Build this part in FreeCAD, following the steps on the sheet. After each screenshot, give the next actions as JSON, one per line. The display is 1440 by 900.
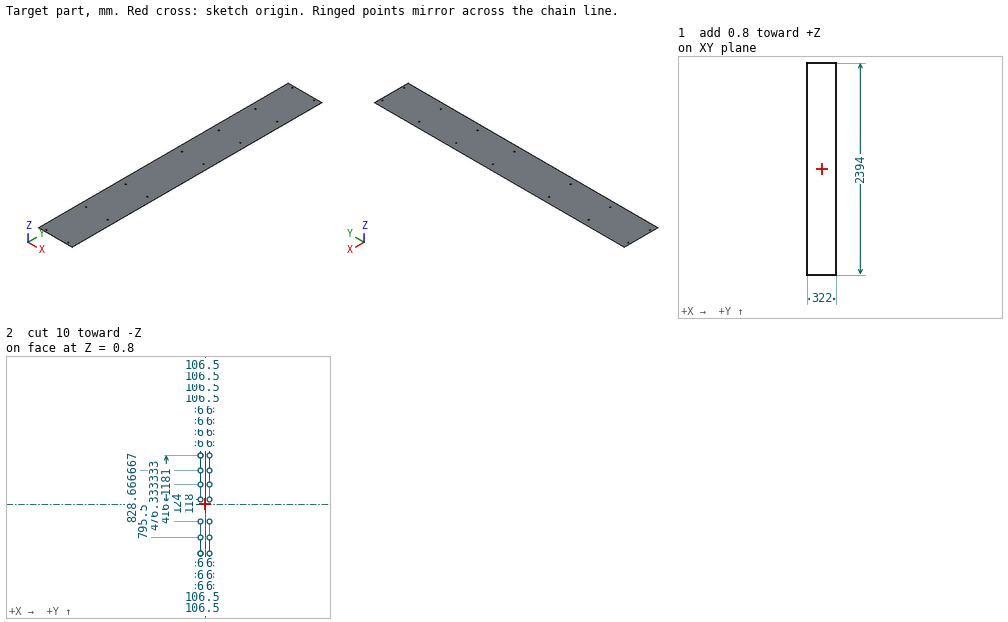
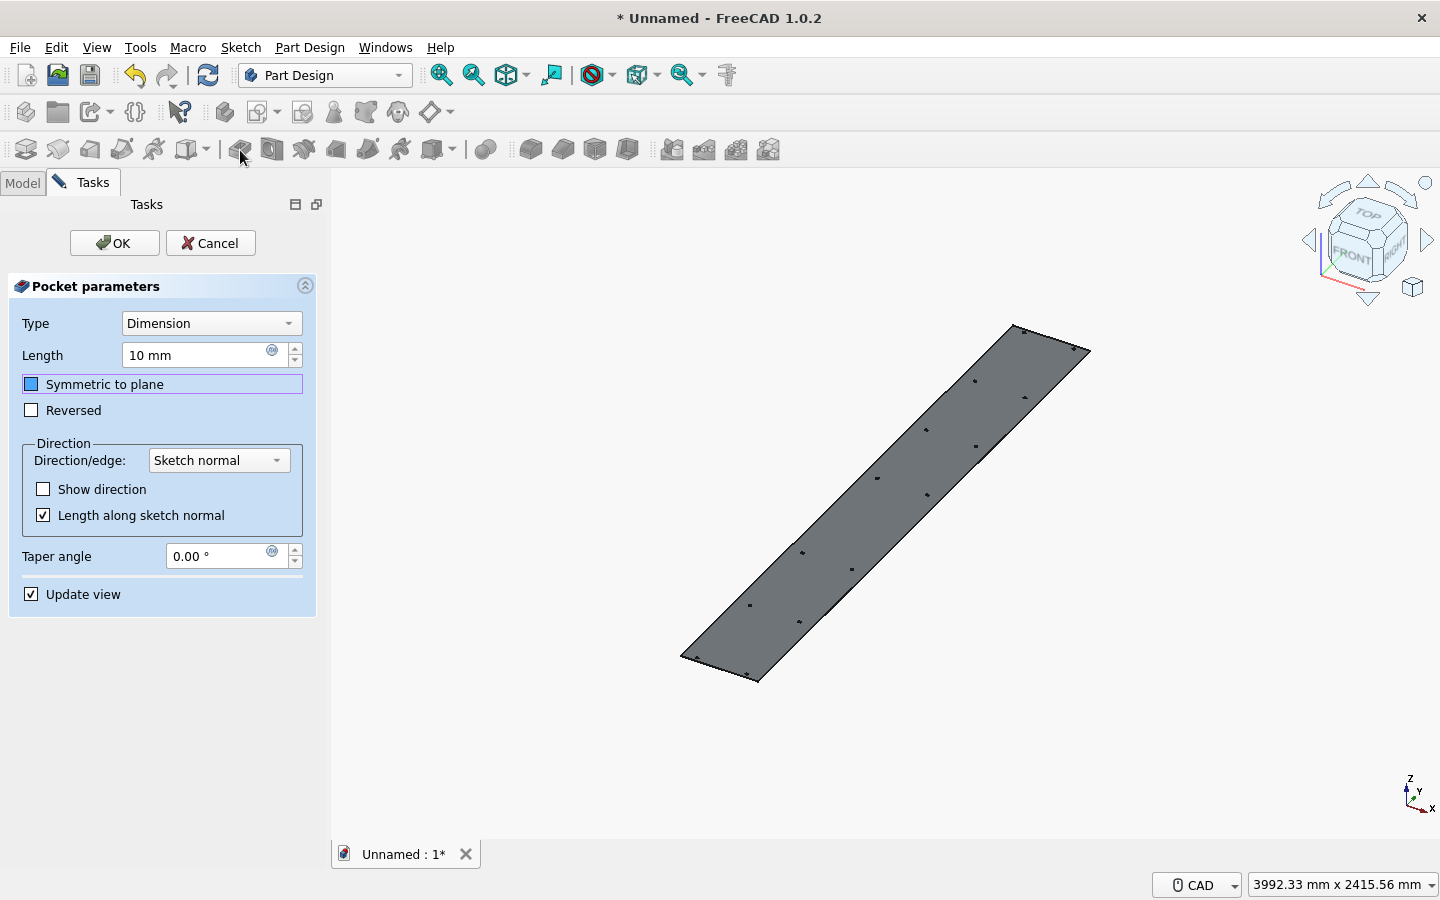
{"action": "left_click", "coordinate": [115, 243]}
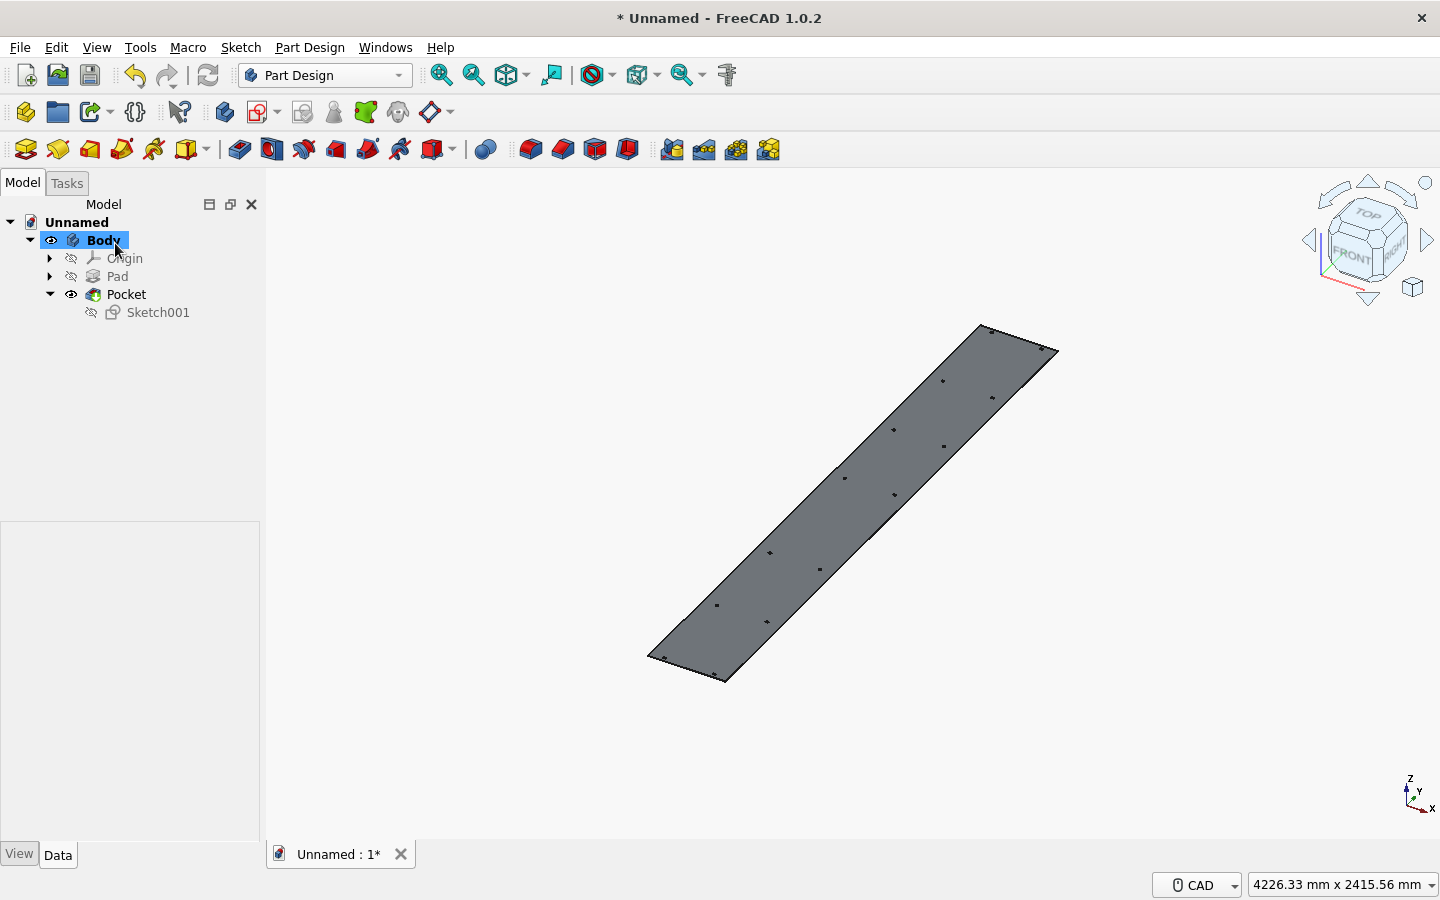
{"action": "key", "text": "0"}